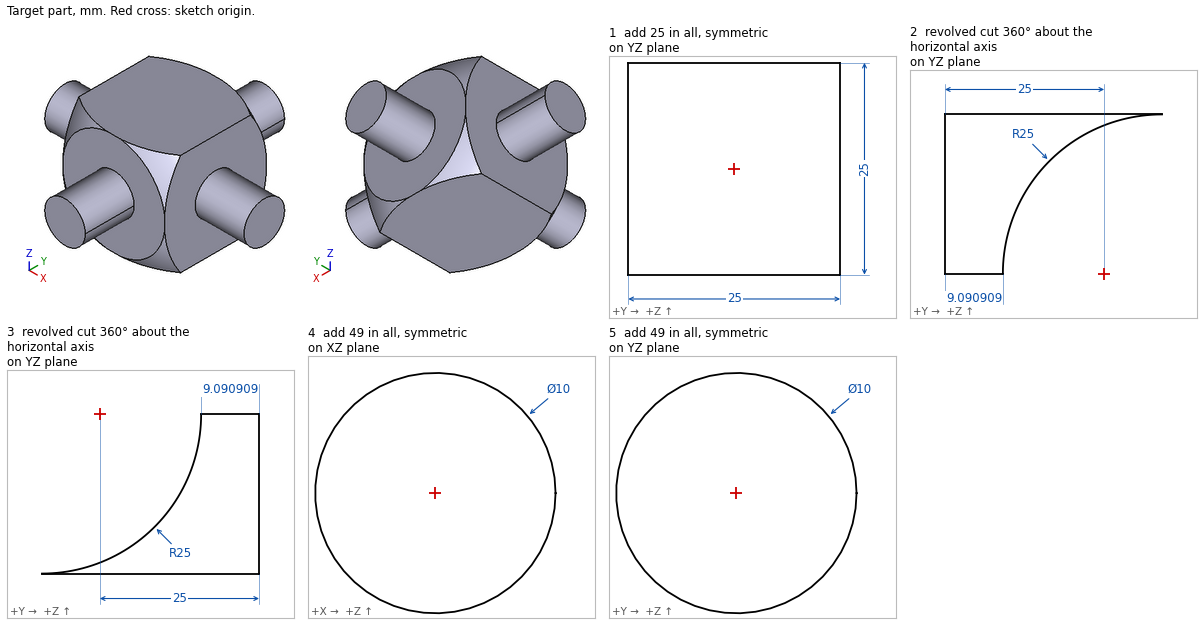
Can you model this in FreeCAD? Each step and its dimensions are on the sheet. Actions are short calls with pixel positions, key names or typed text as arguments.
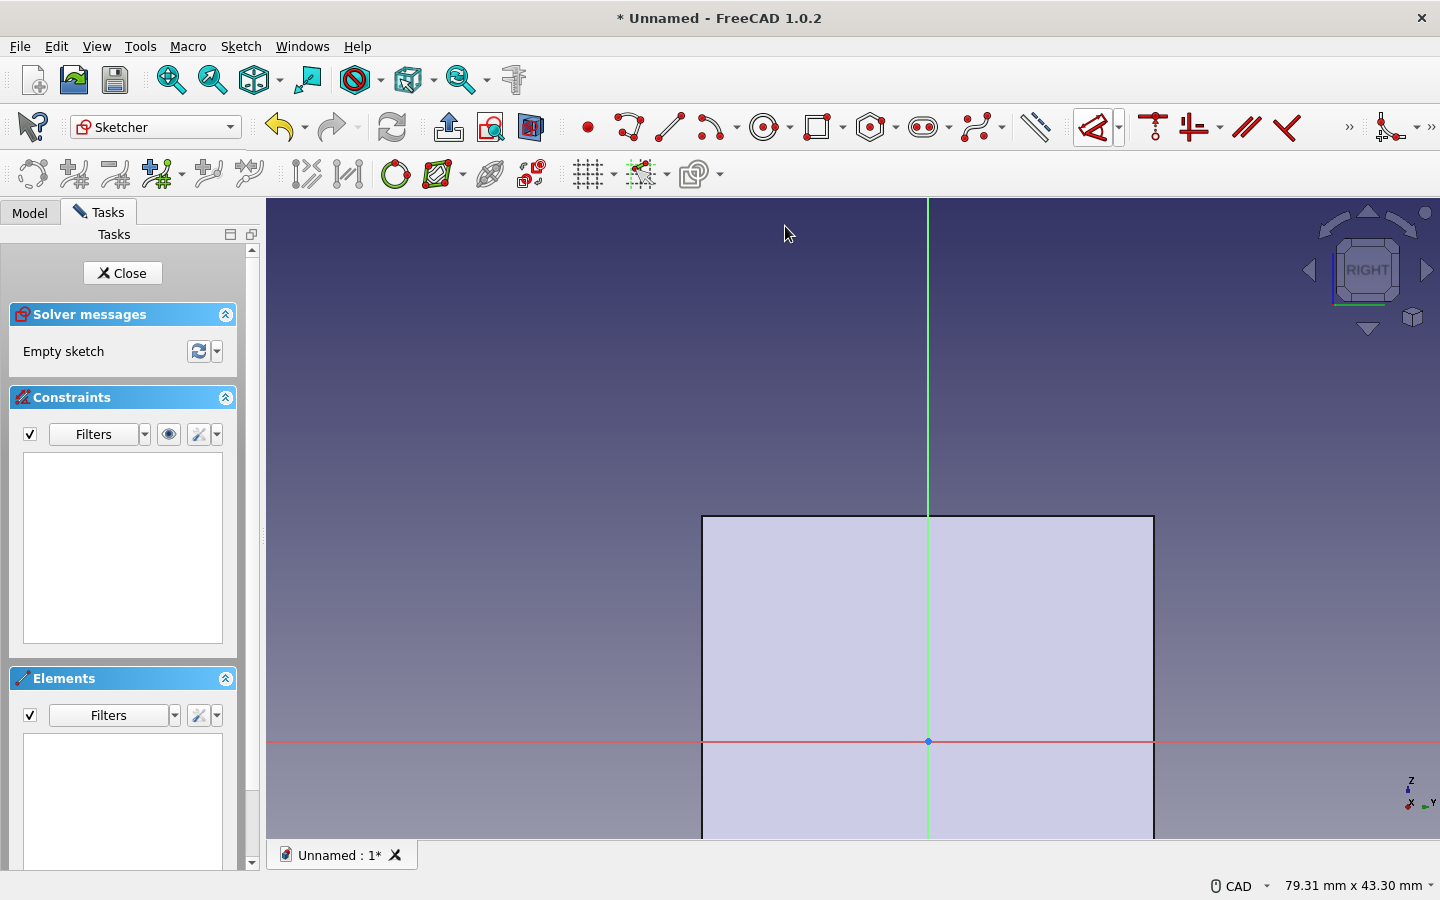
key(g)
key(m)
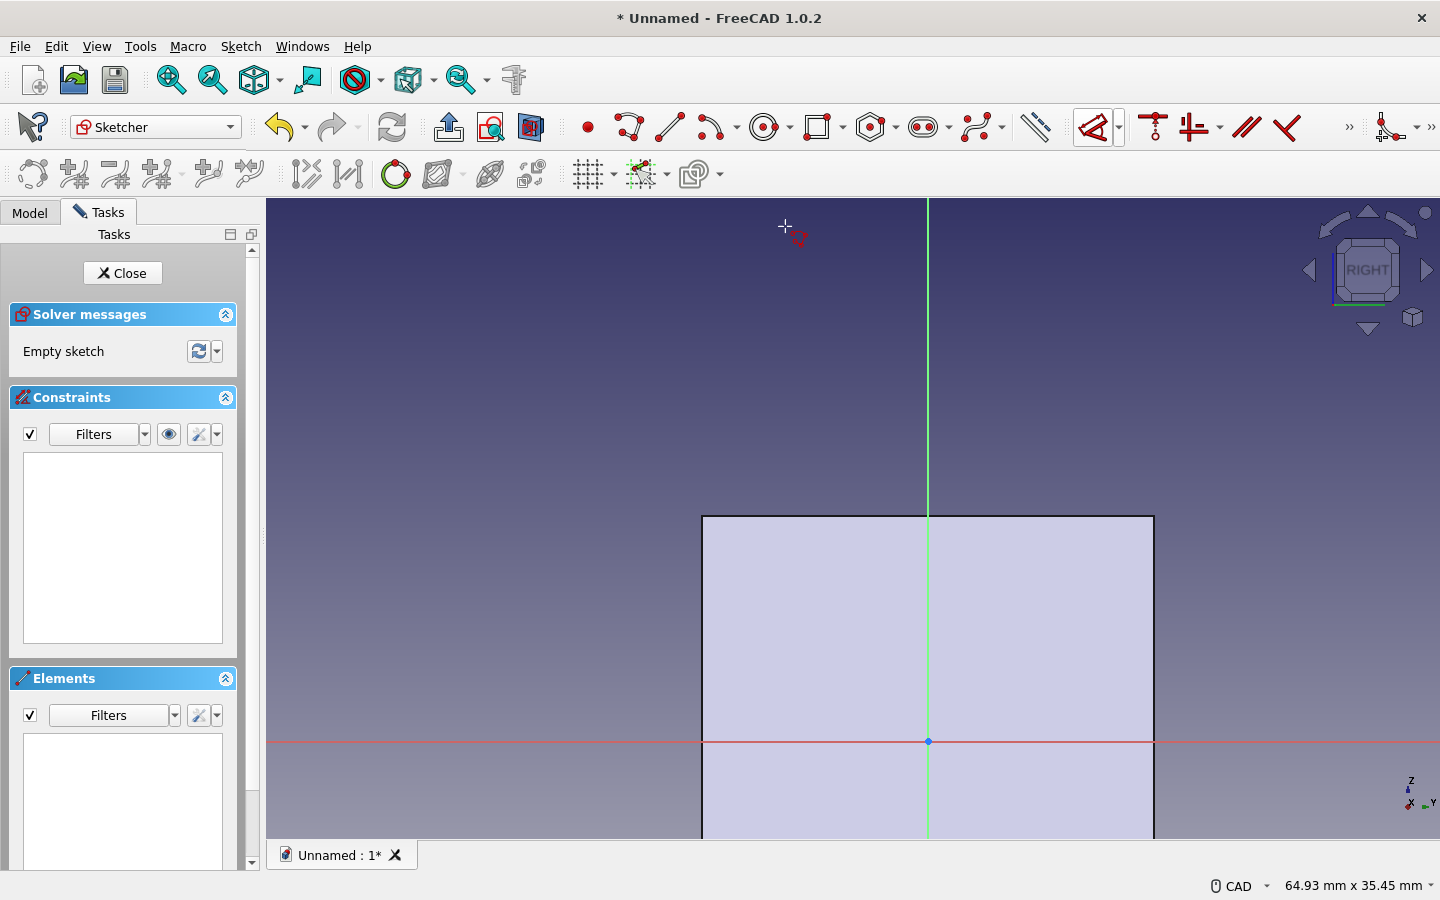
click(1092, 290)
click(476, 290)
click(476, 742)
click(640, 733)
right_click(640, 733)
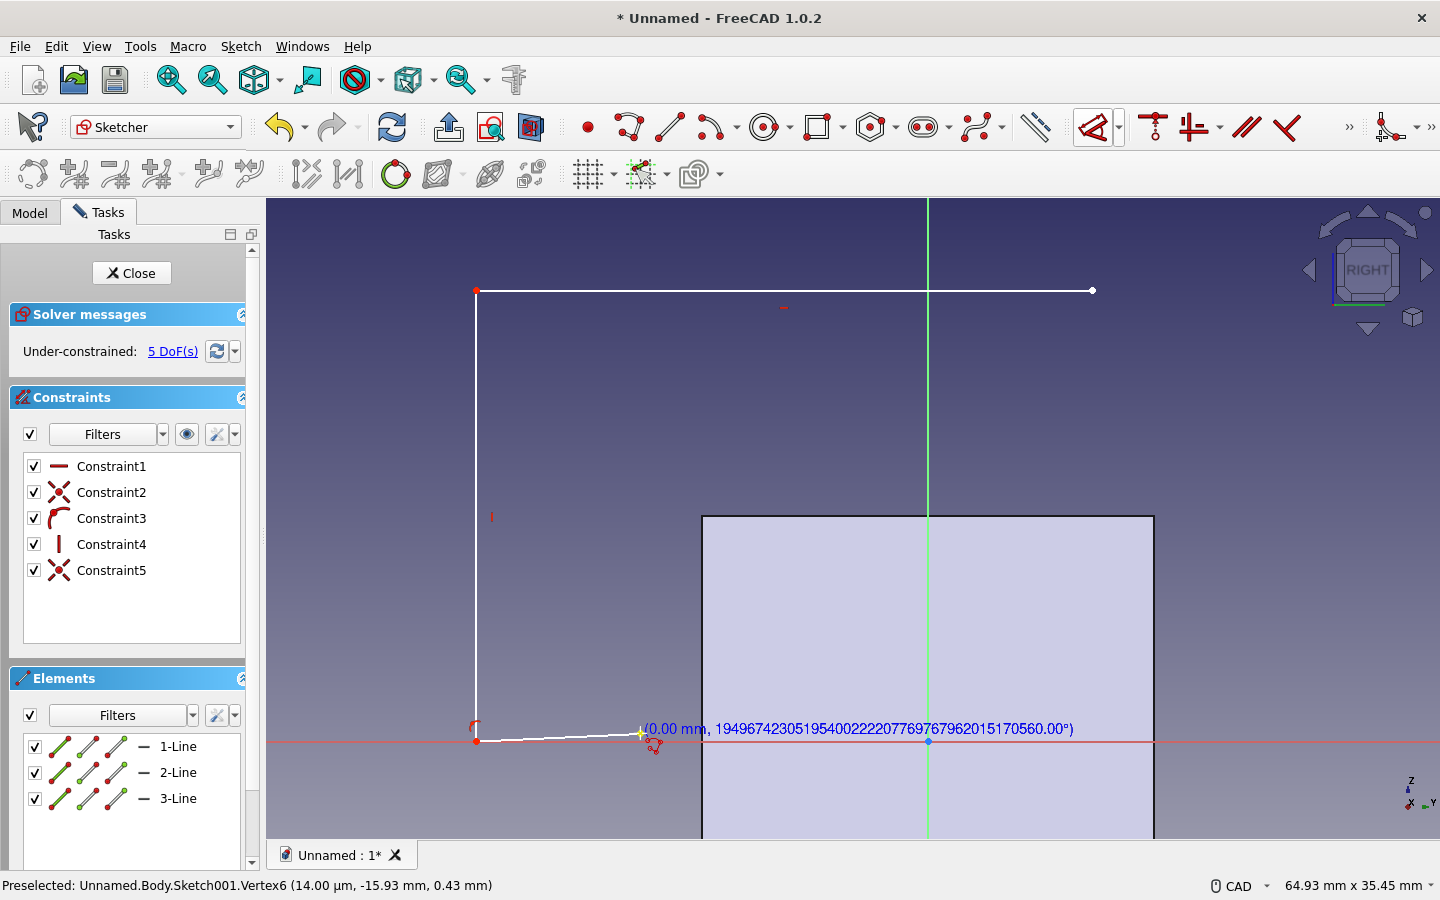
key(g)
key(3)
key(a)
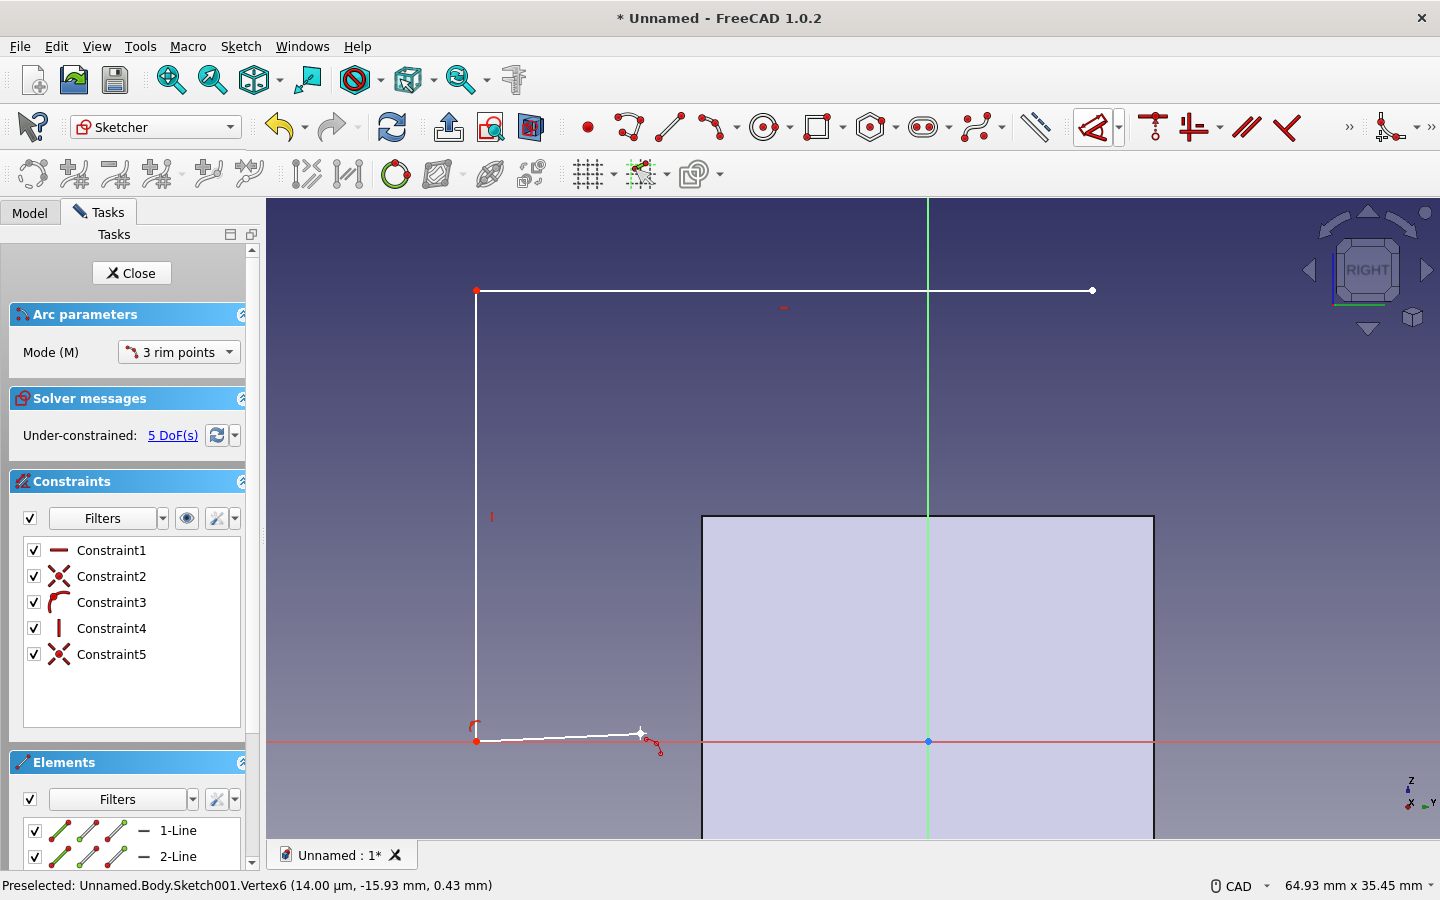
click(640, 734)
click(1092, 291)
click(773, 422)
key(Escape)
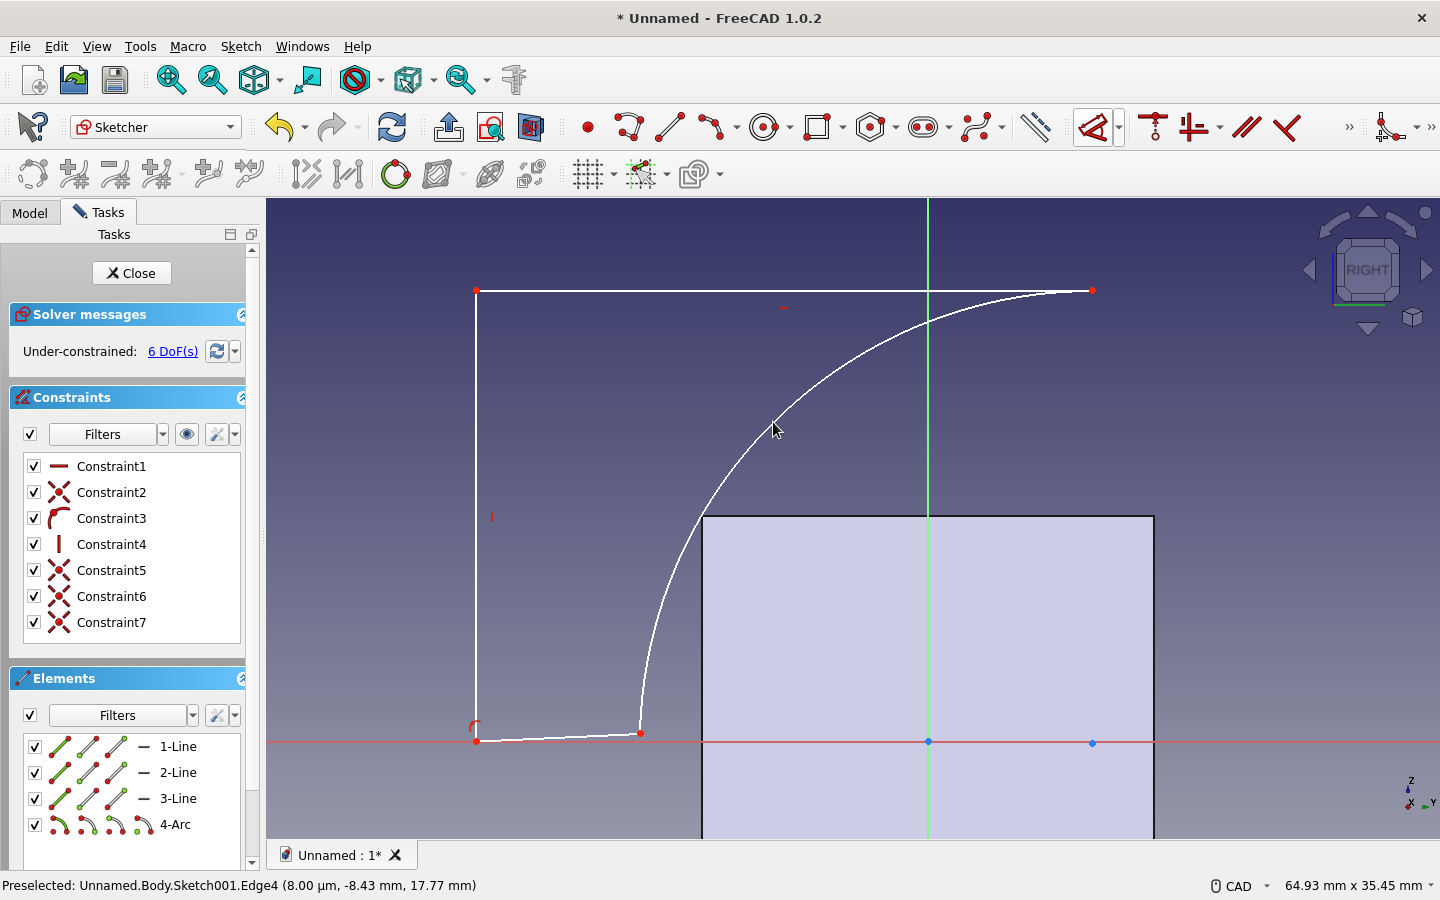
click(907, 291)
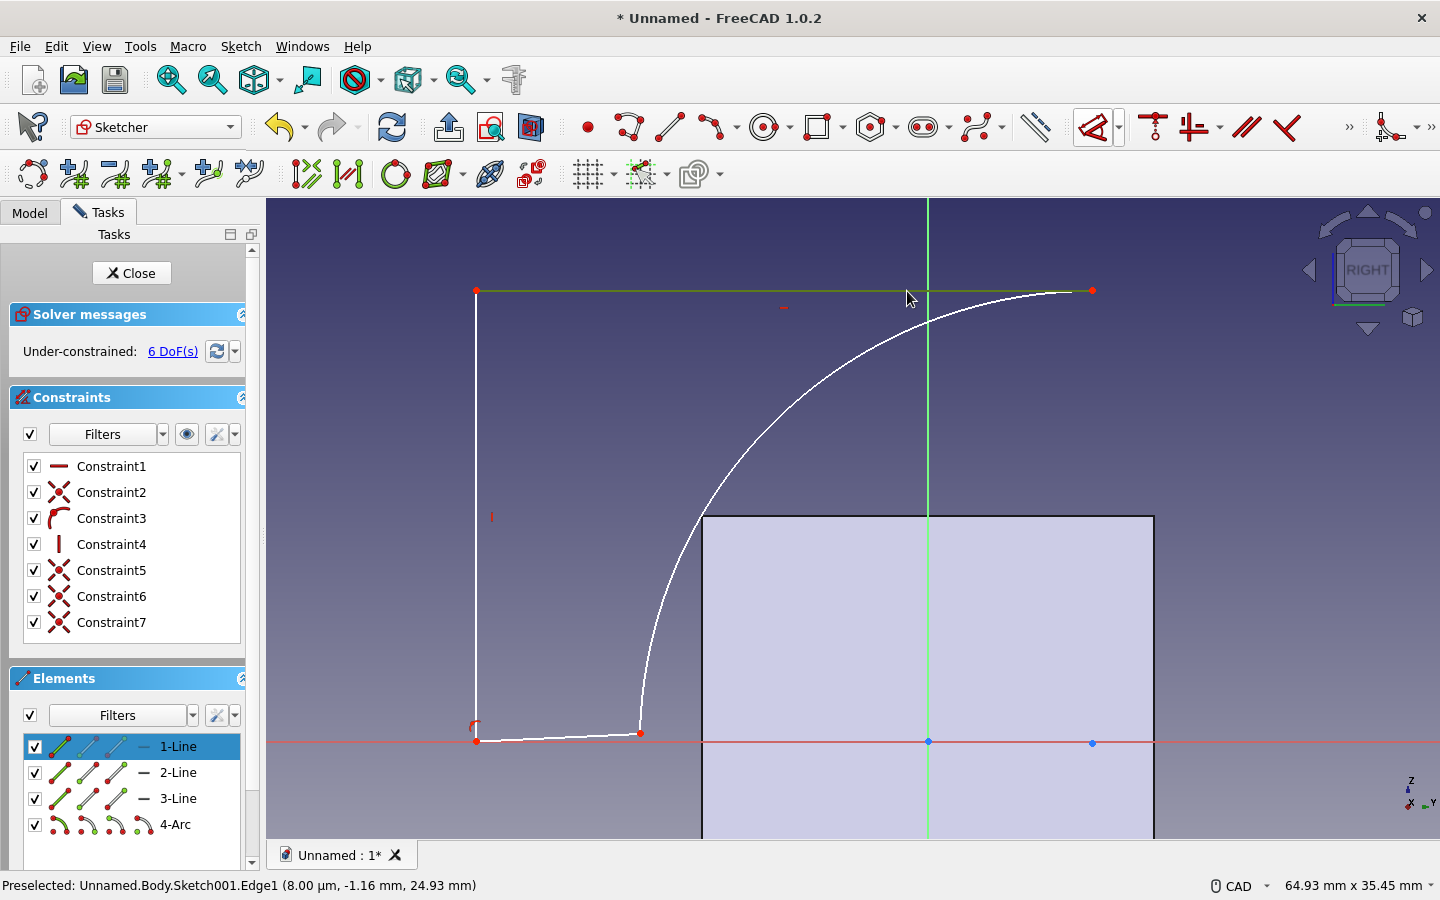
click(889, 339)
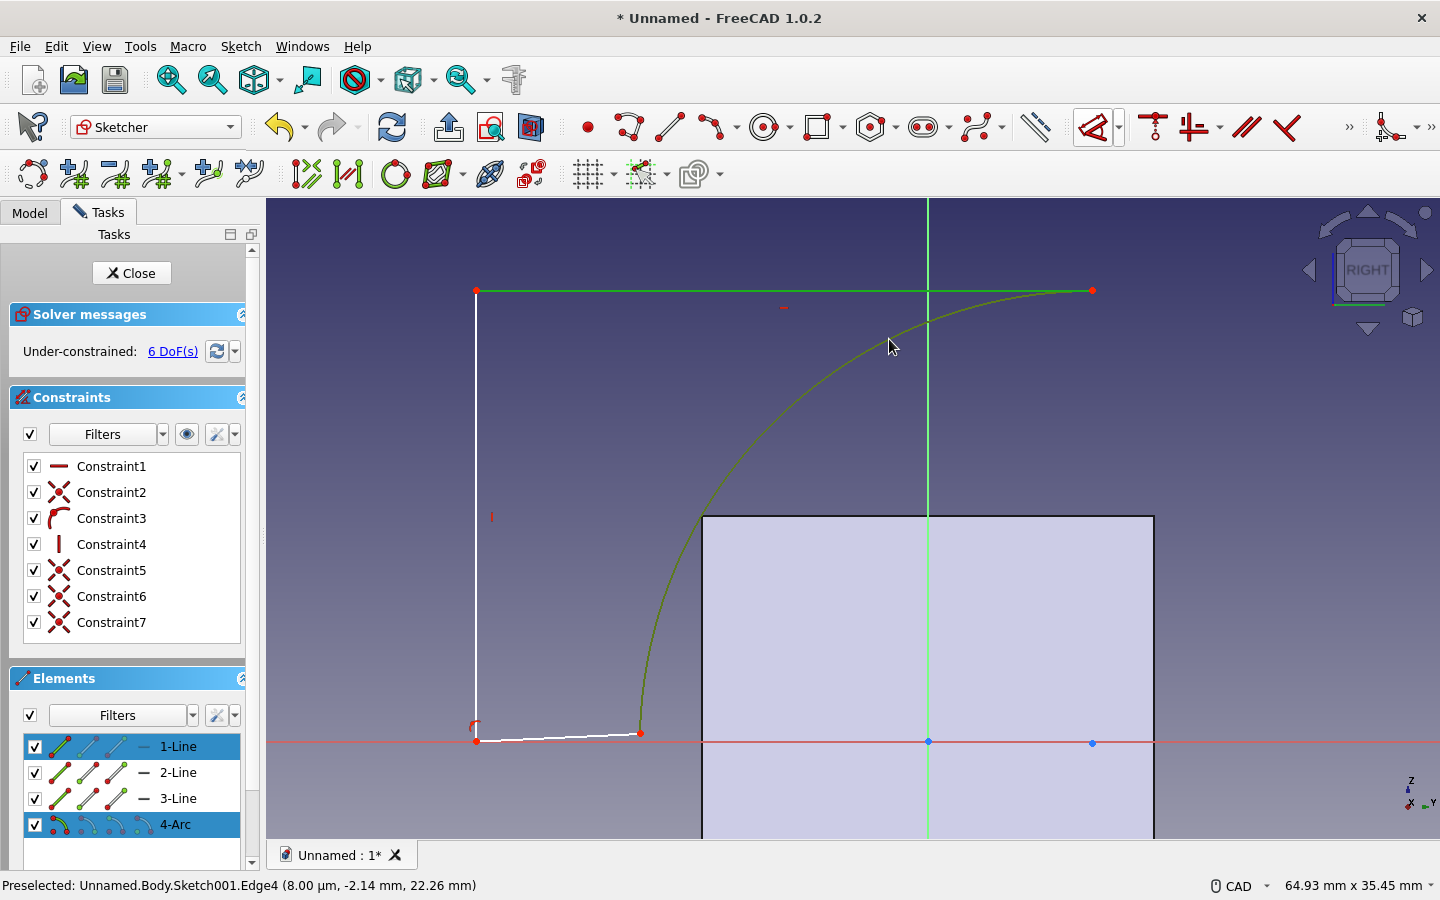
key(t)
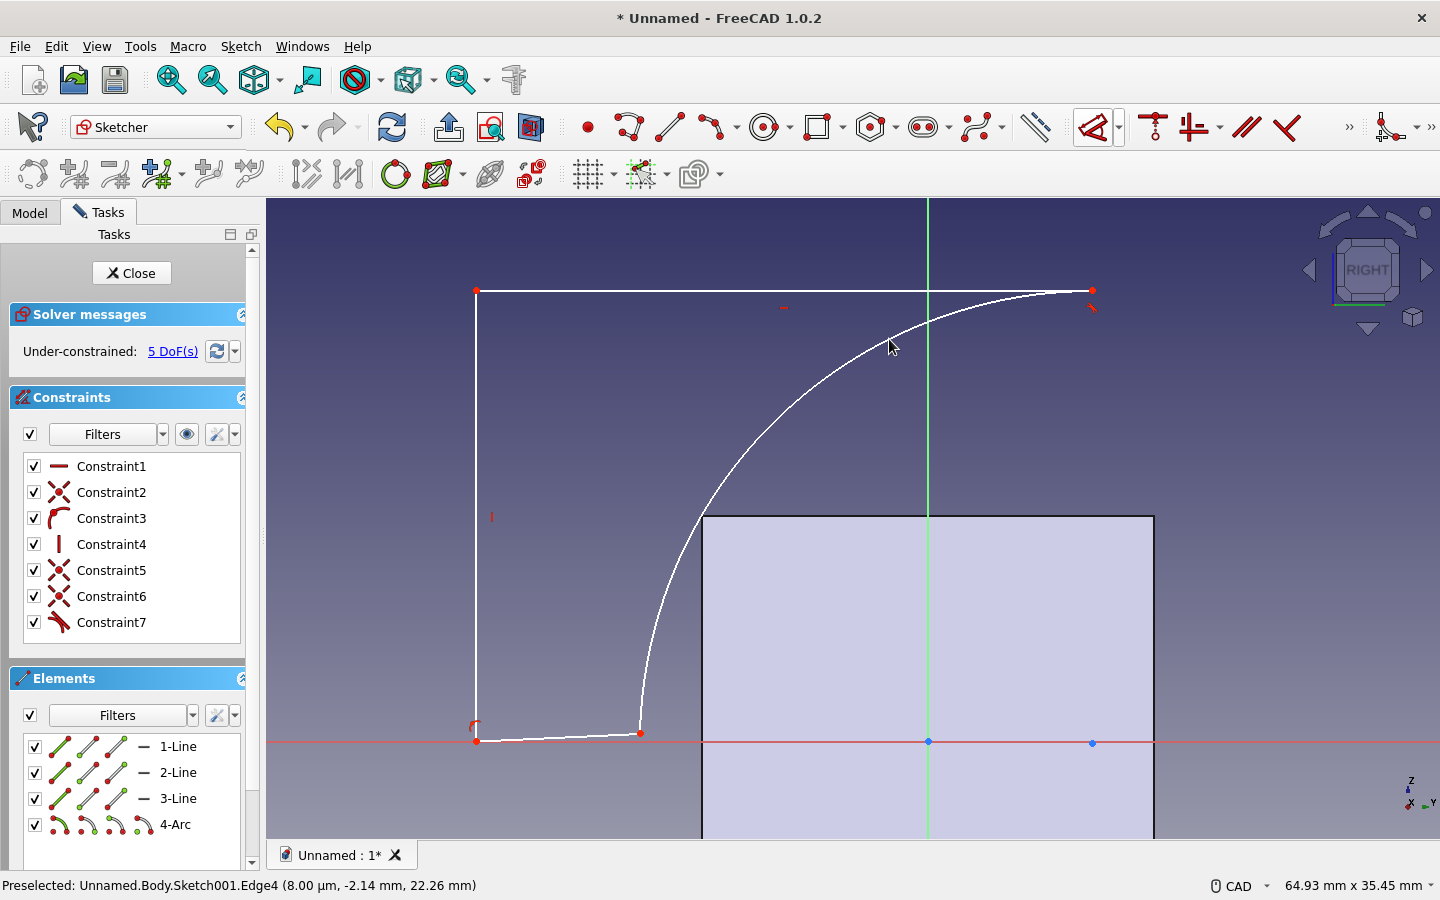
click(525, 739)